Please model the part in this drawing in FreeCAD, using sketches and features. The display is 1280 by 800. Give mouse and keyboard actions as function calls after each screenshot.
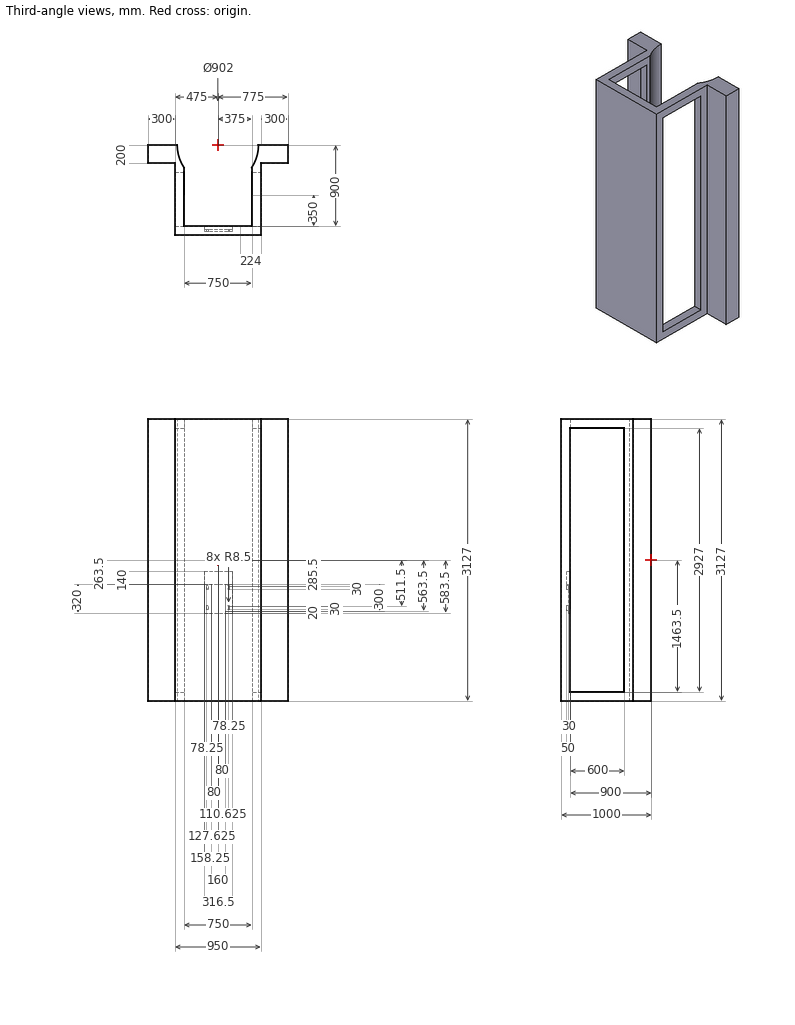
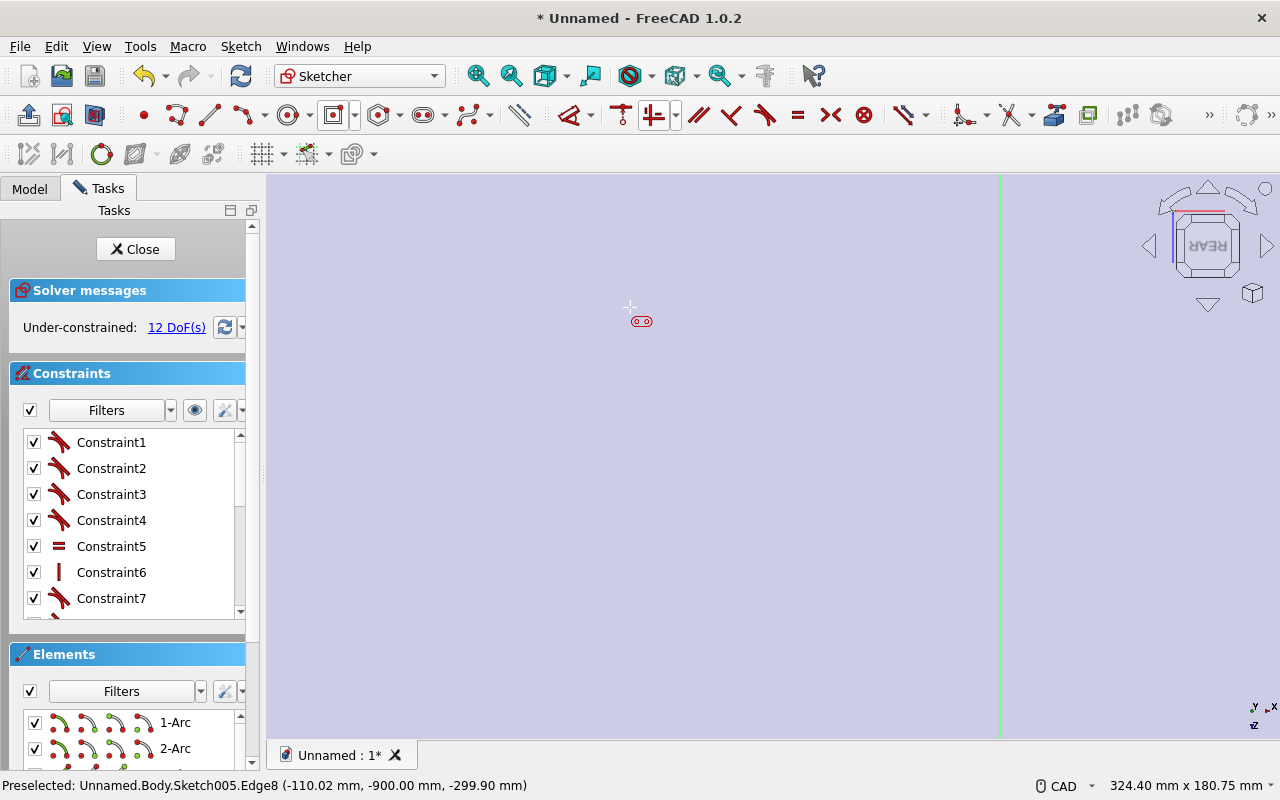
scroll(630, 307, down, 8)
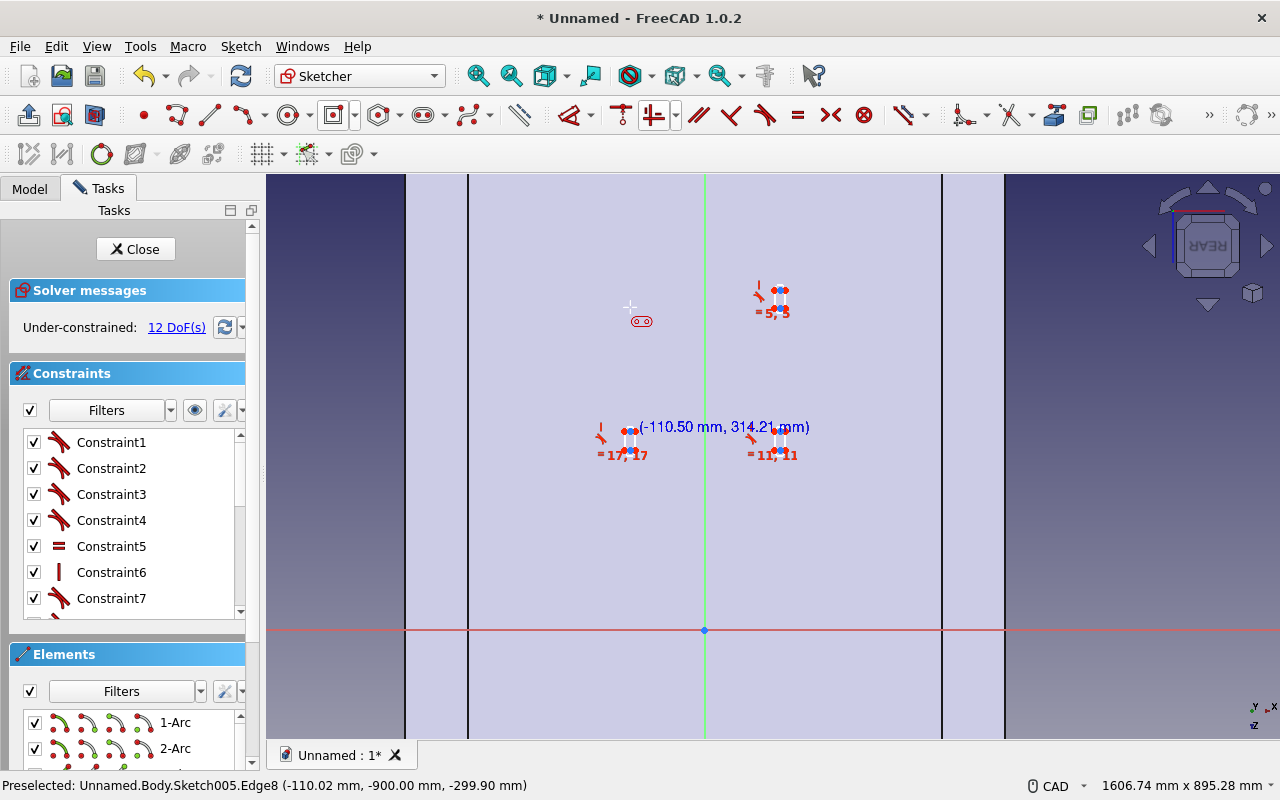
click(630, 307)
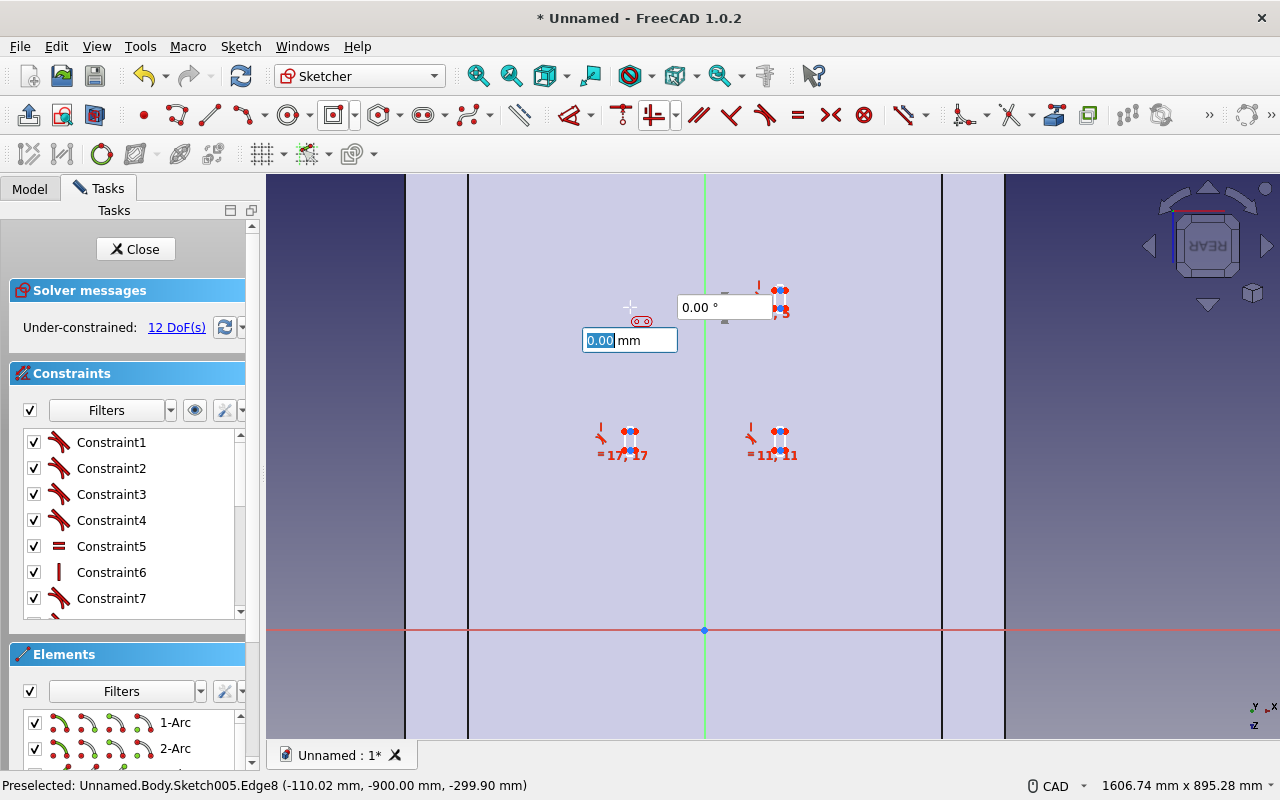
click(630, 289)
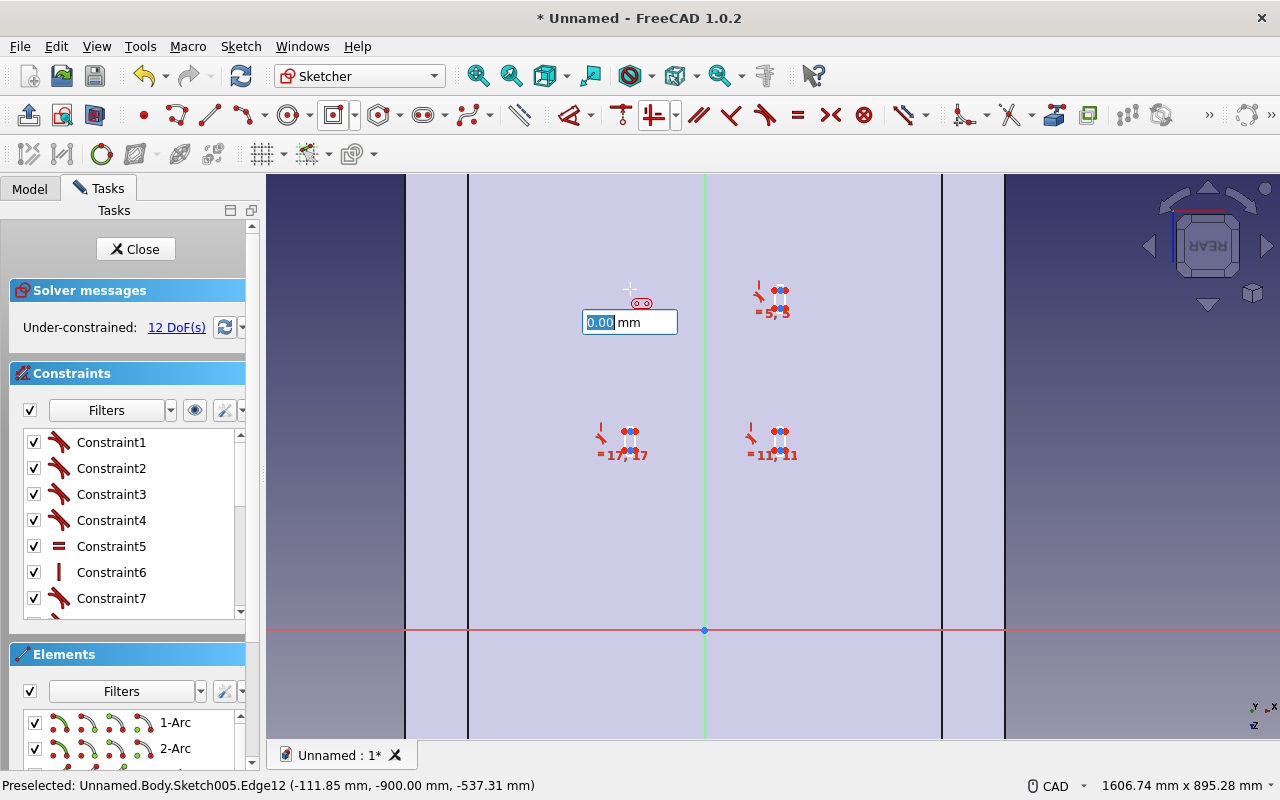
scroll(624, 298, up, 6)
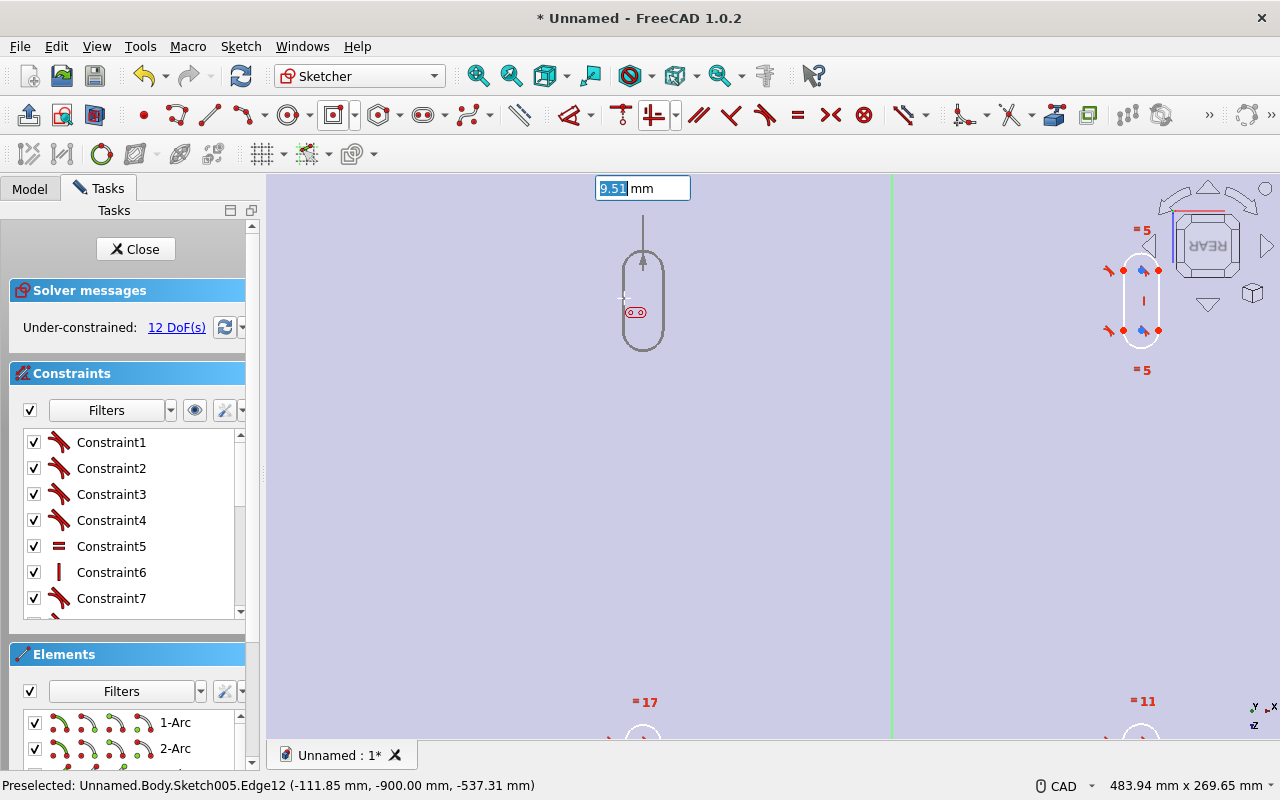
click(625, 298)
key(Escape)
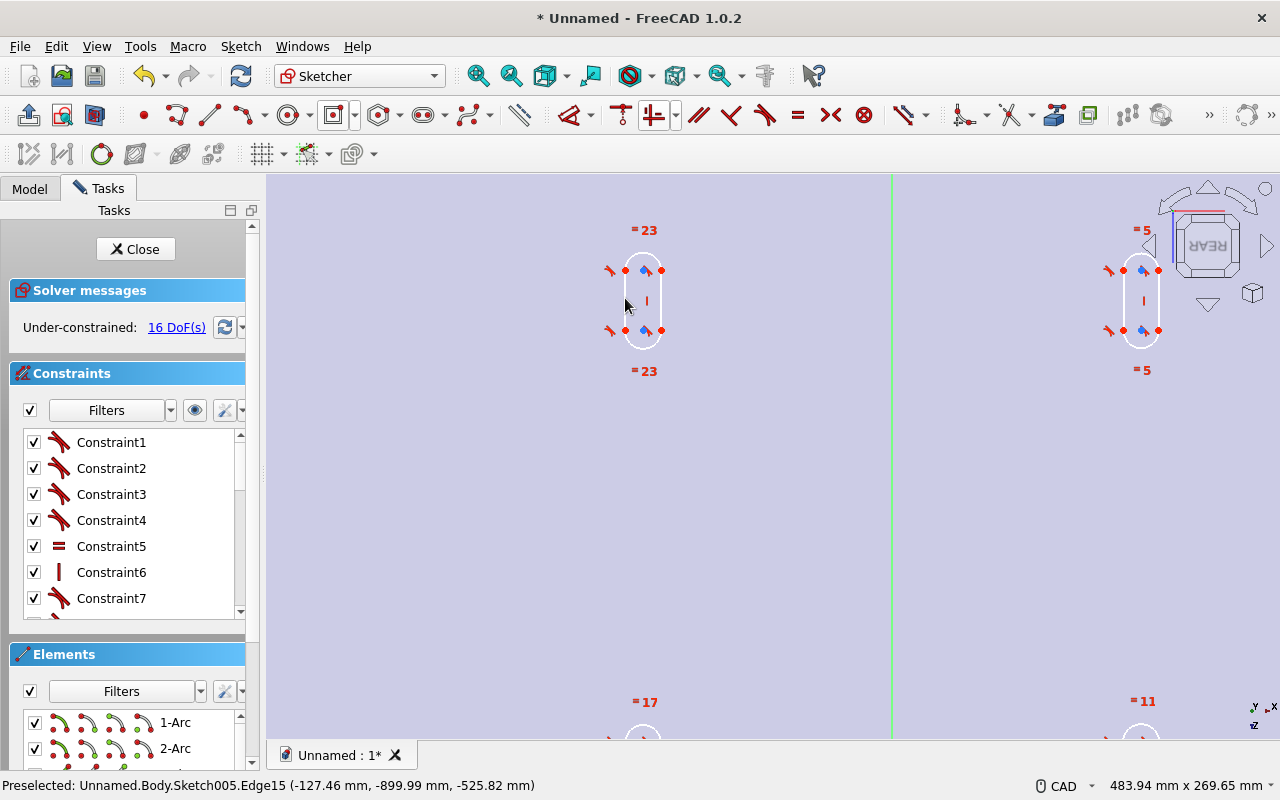
scroll(624, 298, down, 6)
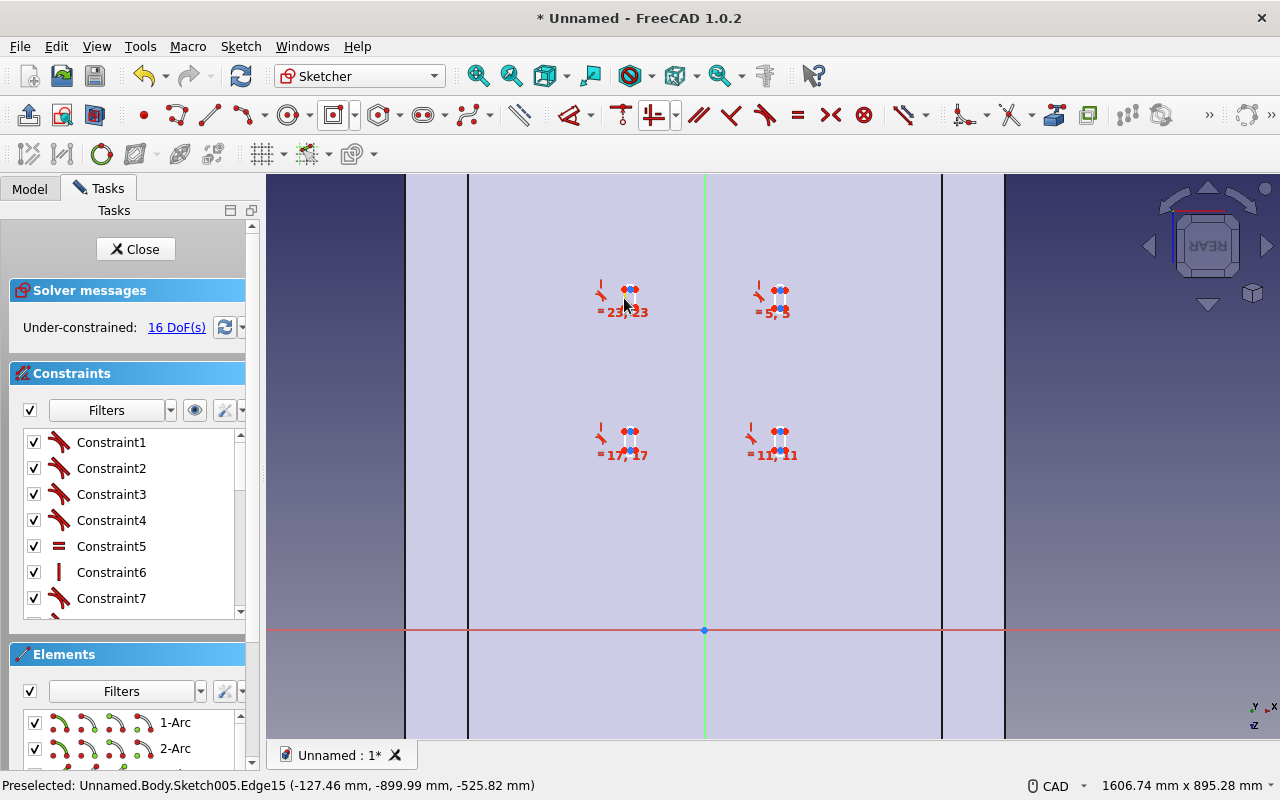
scroll(777, 312, up, 6)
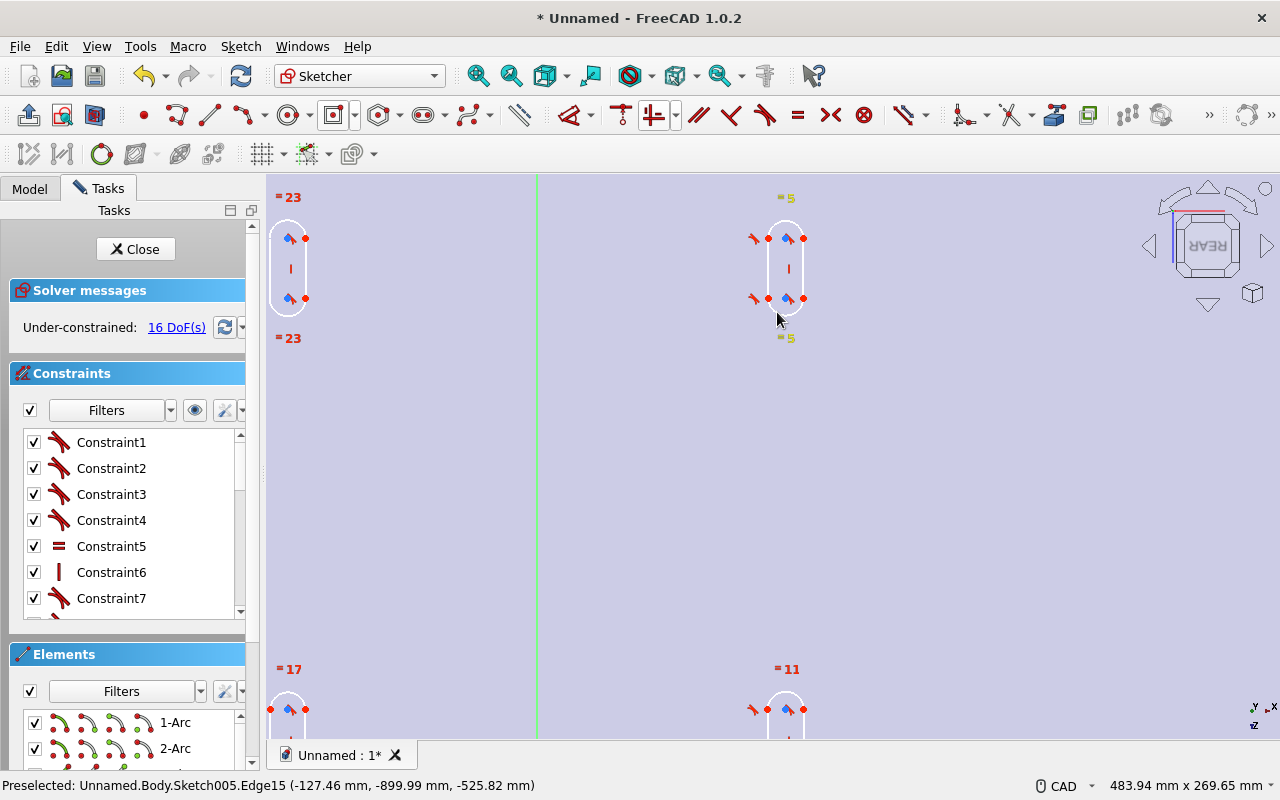
click(776, 312)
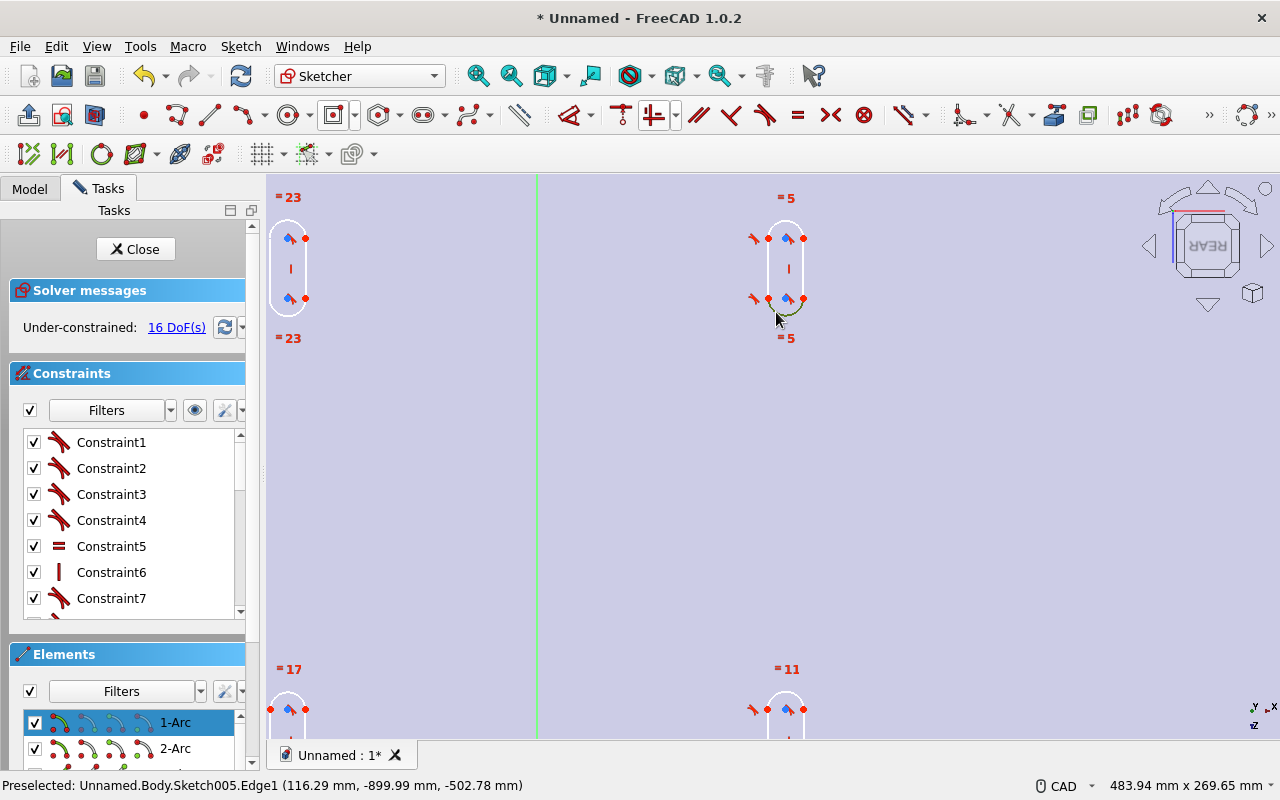
scroll(777, 312, down, 6)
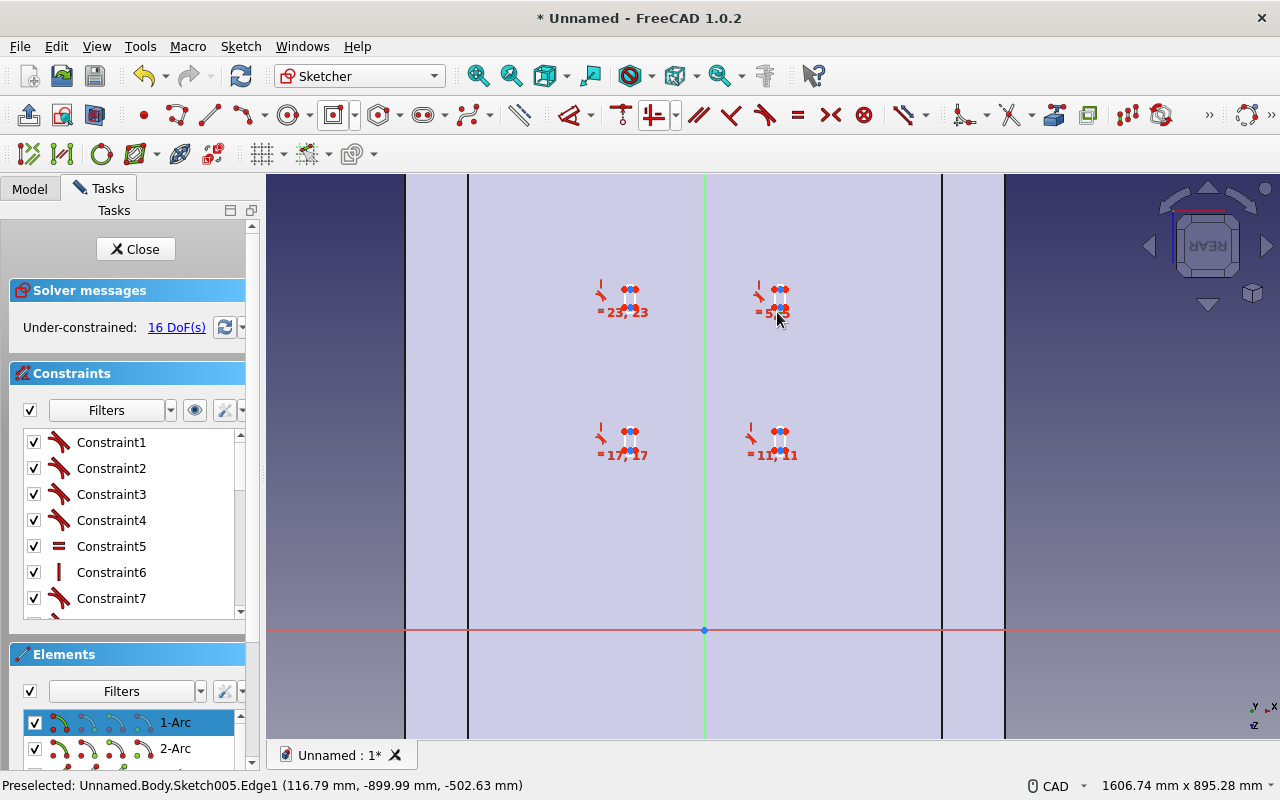
scroll(777, 455, up, 6)